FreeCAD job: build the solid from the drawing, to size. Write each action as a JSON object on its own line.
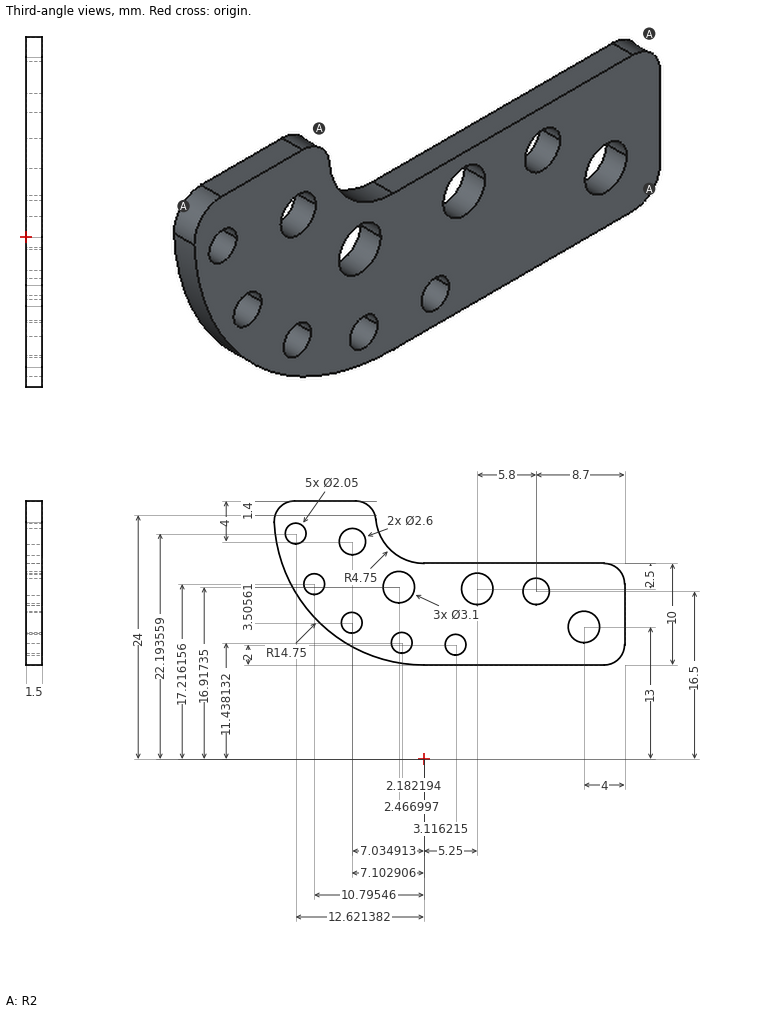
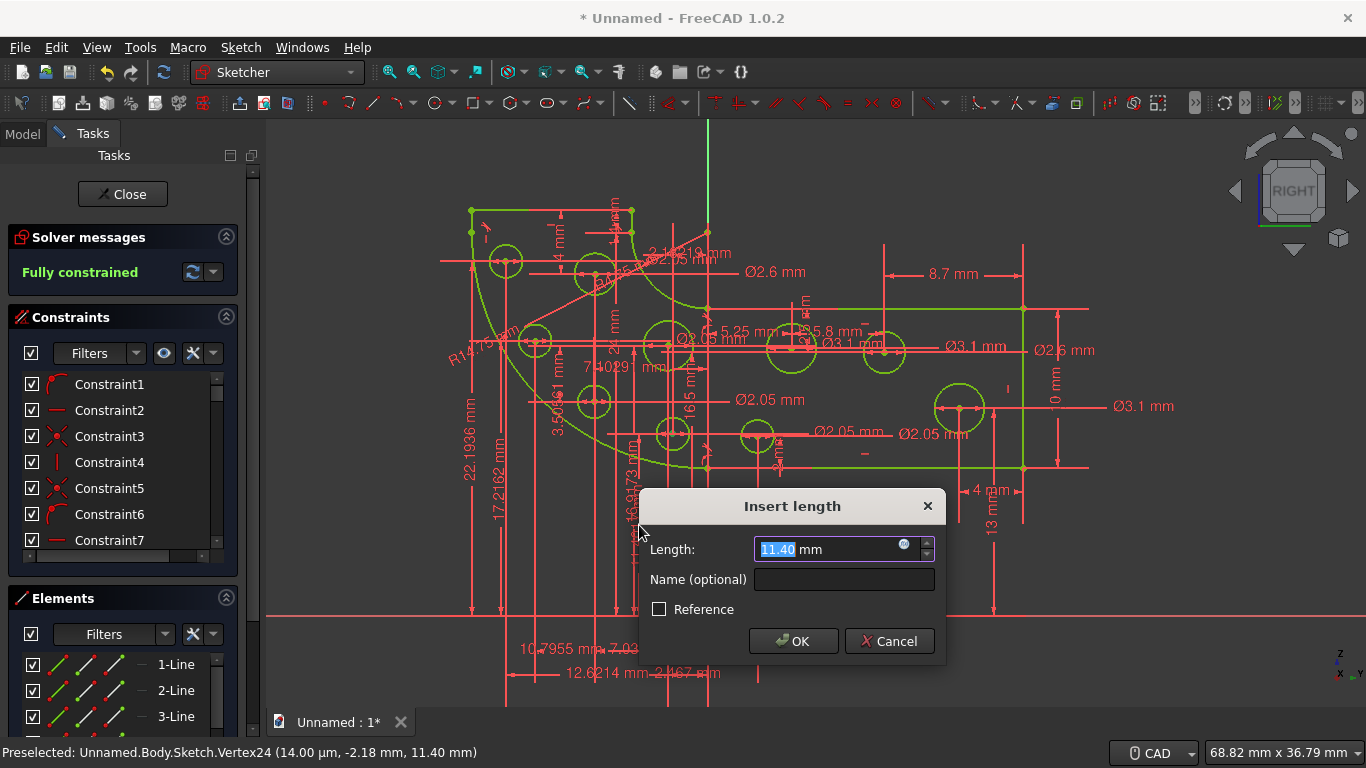
{"action": "type", "text": "11.438132"}
{"action": "key", "text": "Return"}
{"action": "key", "text": "Escape"}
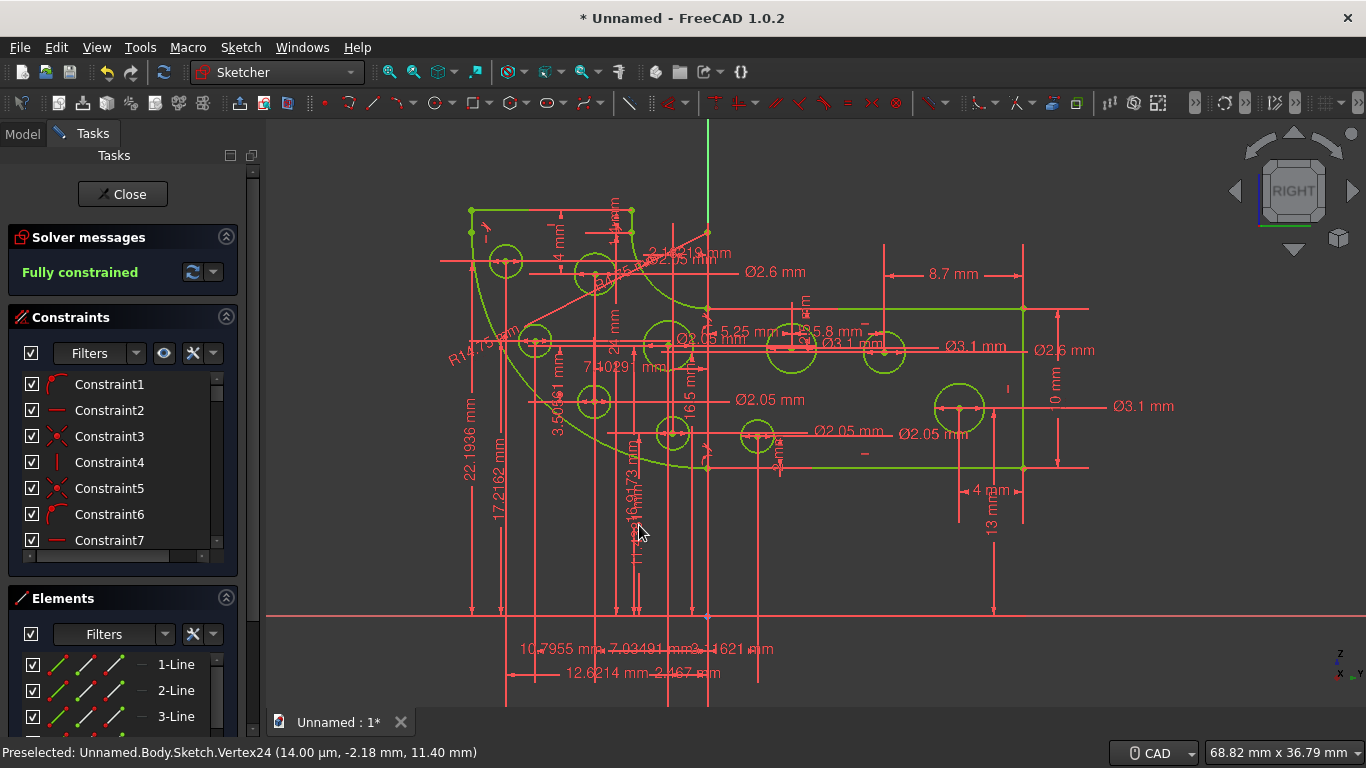
{"action": "left_click", "coordinate": [123, 194]}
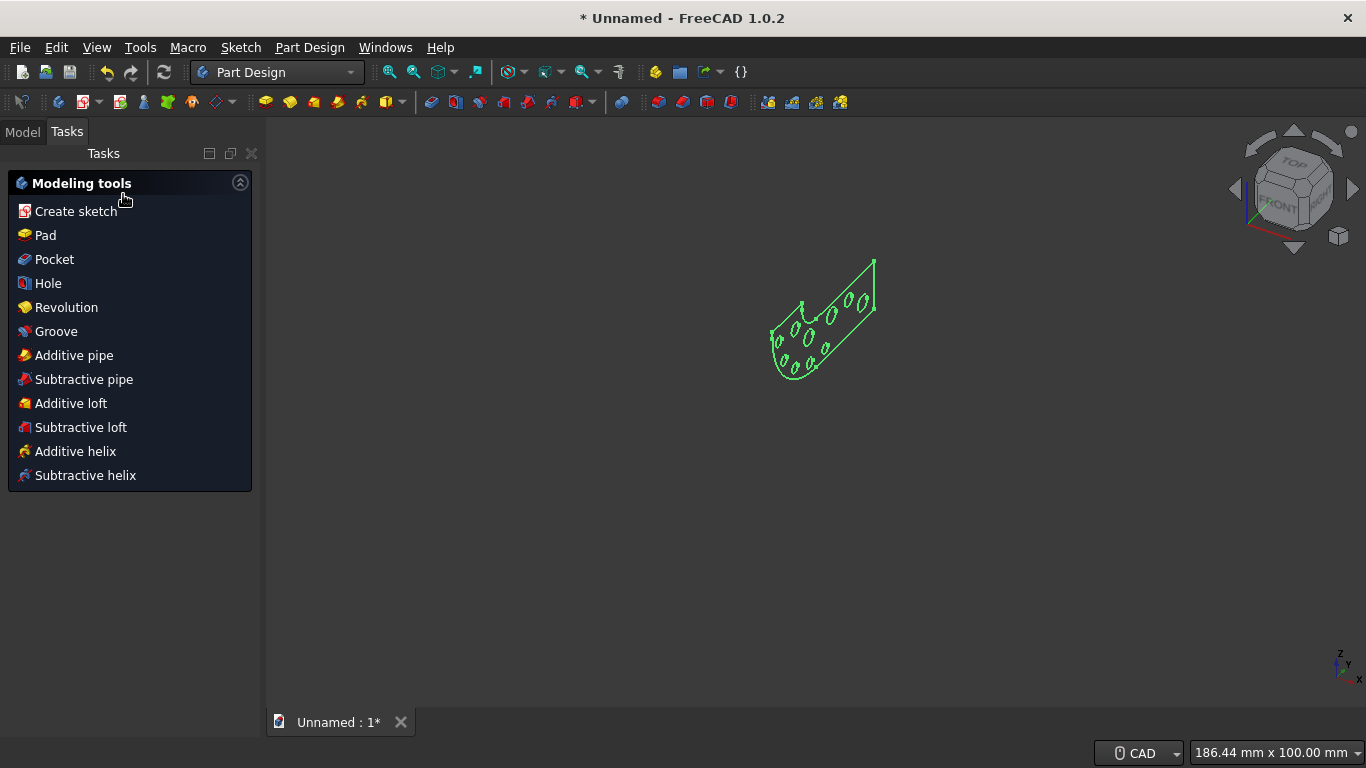
{"action": "left_click", "coordinate": [266, 102]}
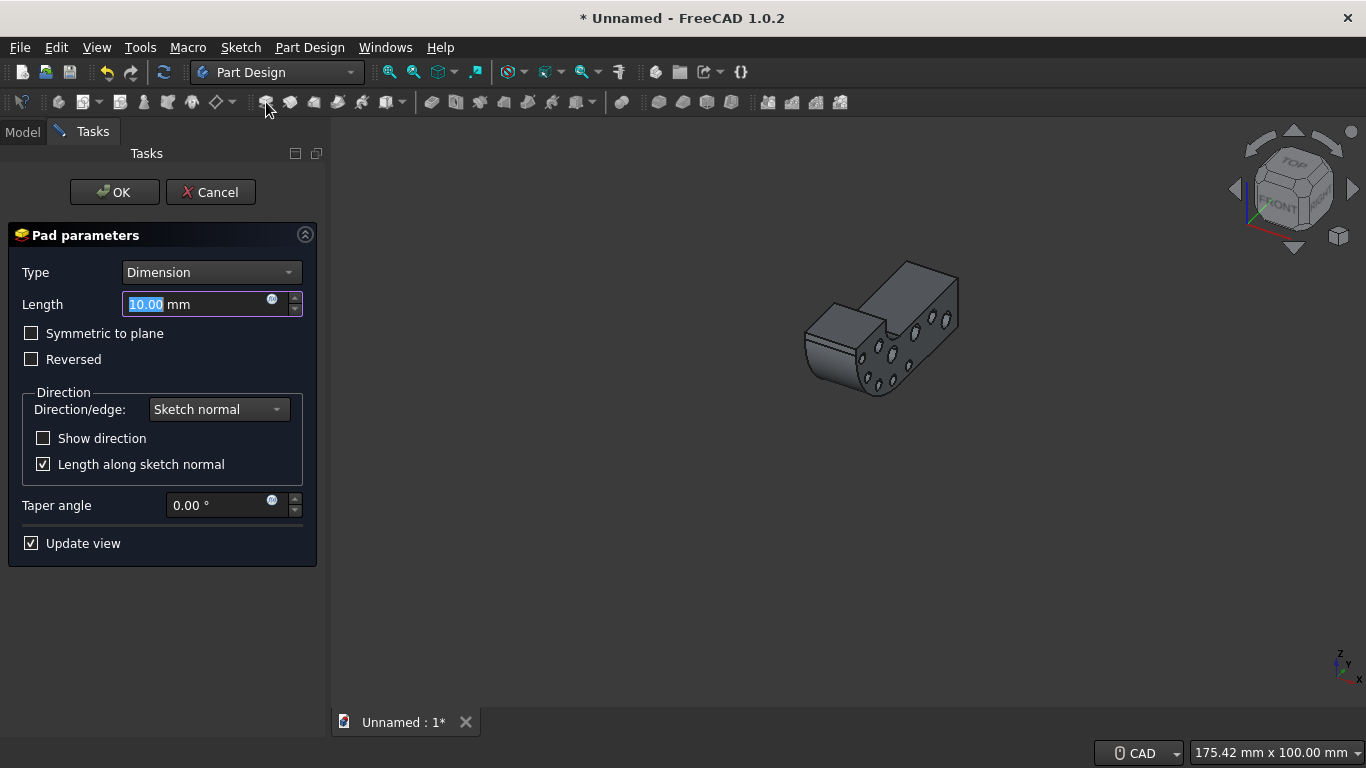
{"action": "type", "text": "1.5"}
{"action": "key", "text": "Tab"}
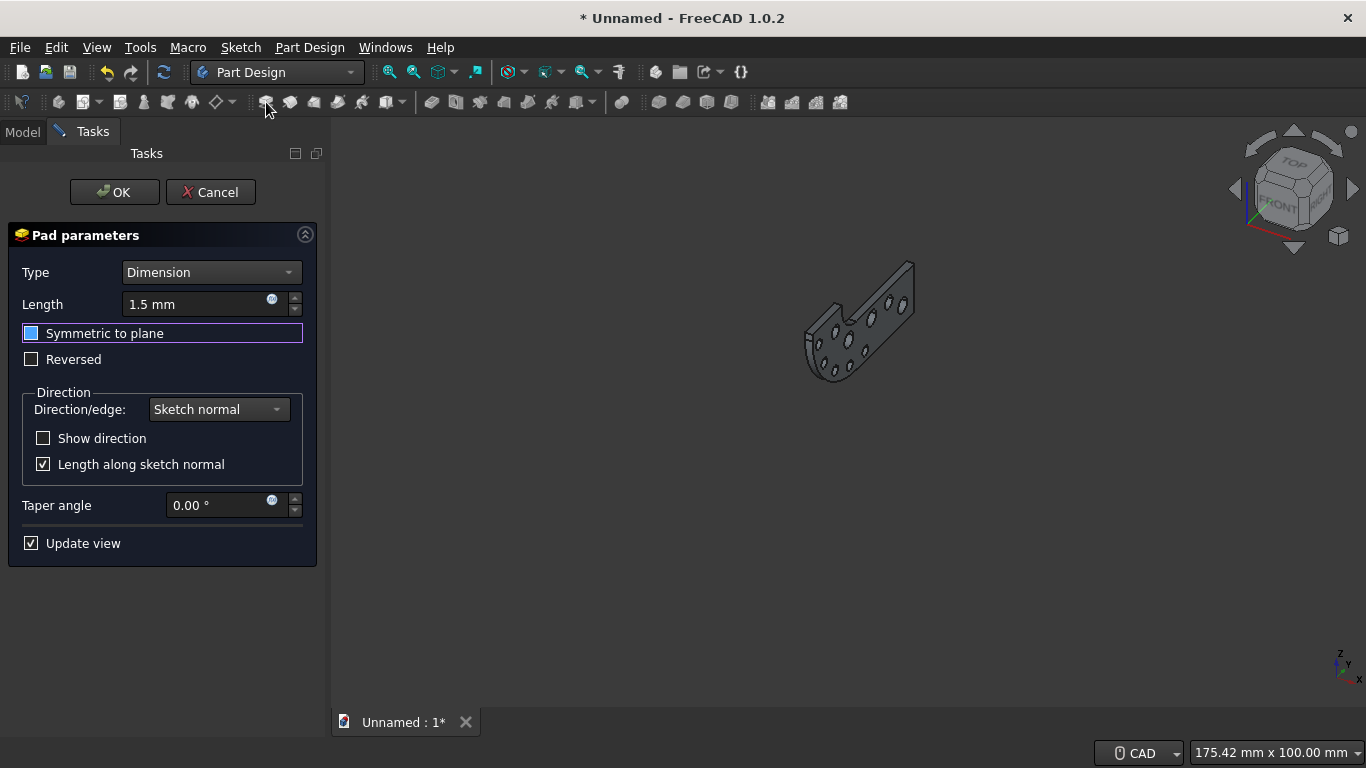
{"action": "left_click", "coordinate": [115, 192]}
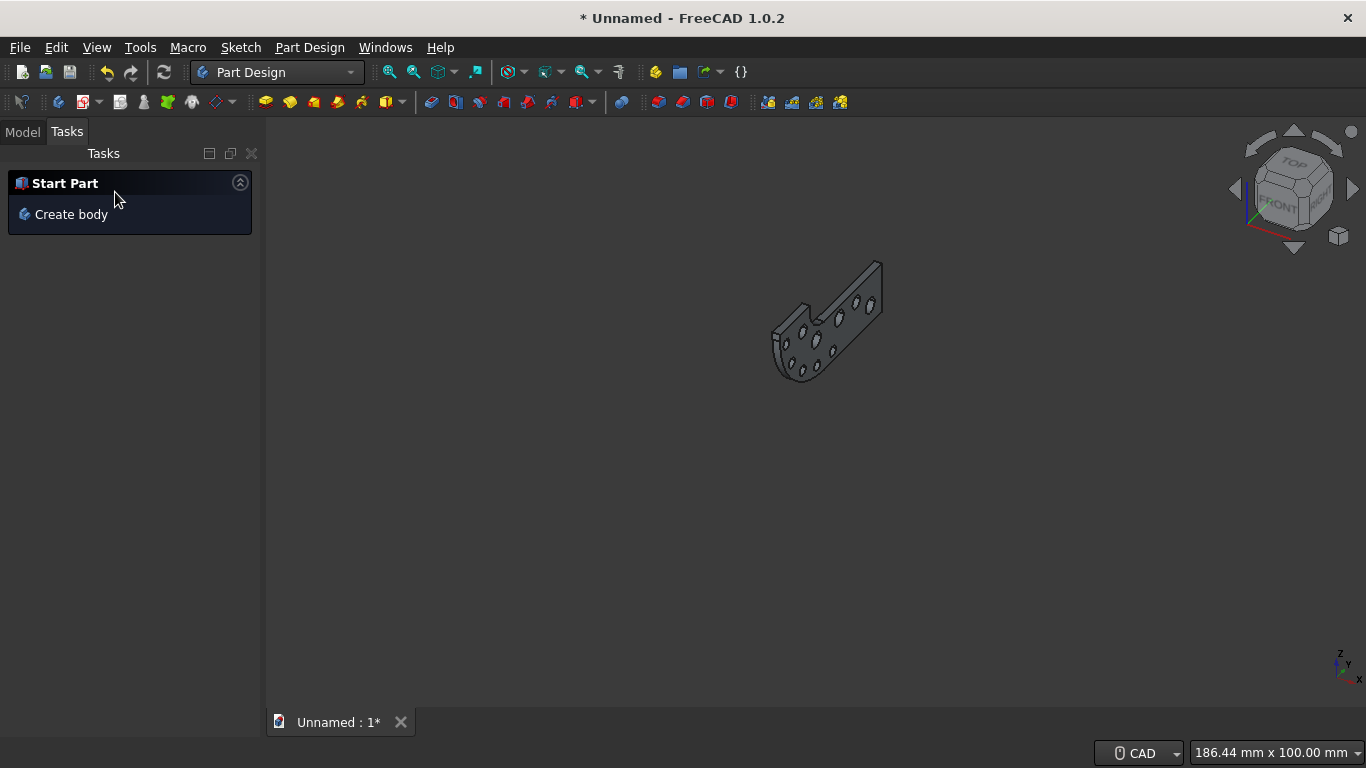
{"action": "key", "text": "v f"}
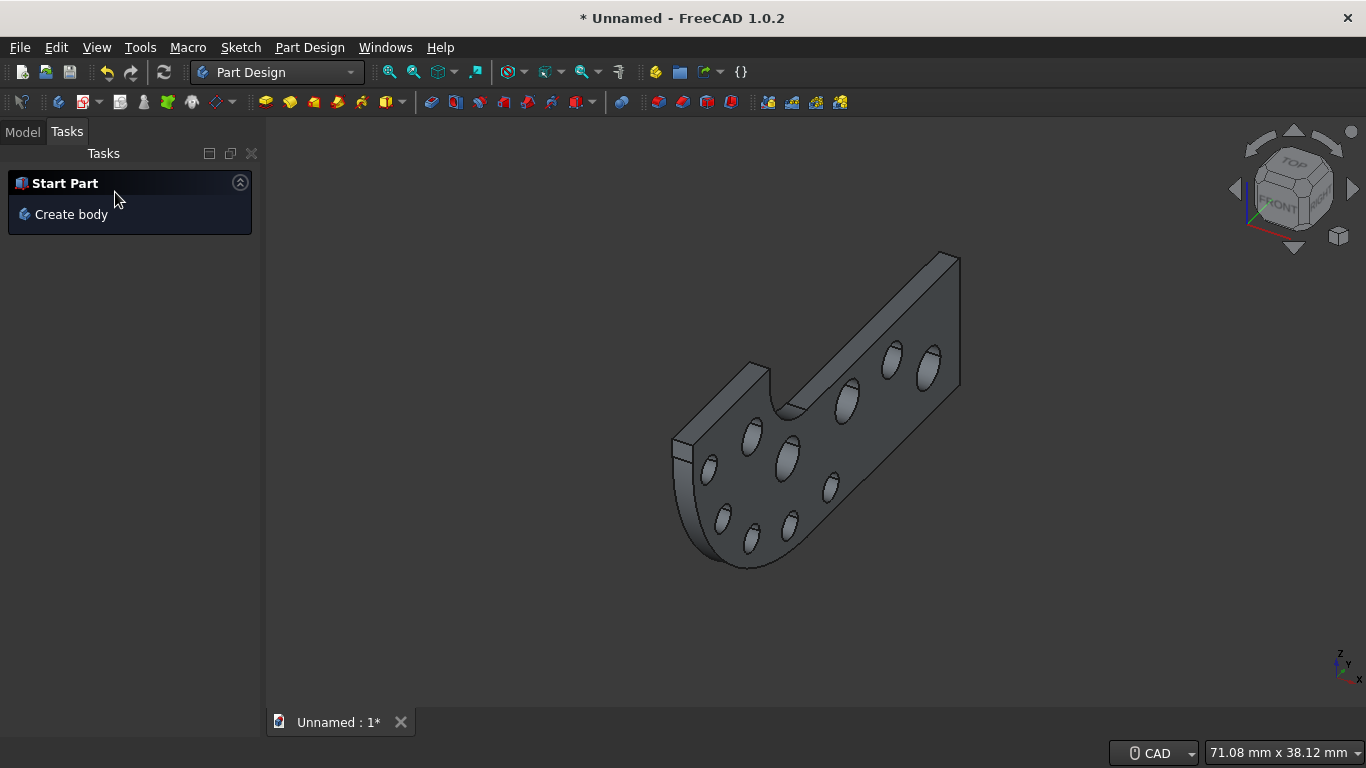
{"action": "left_click", "coordinate": [683, 441]}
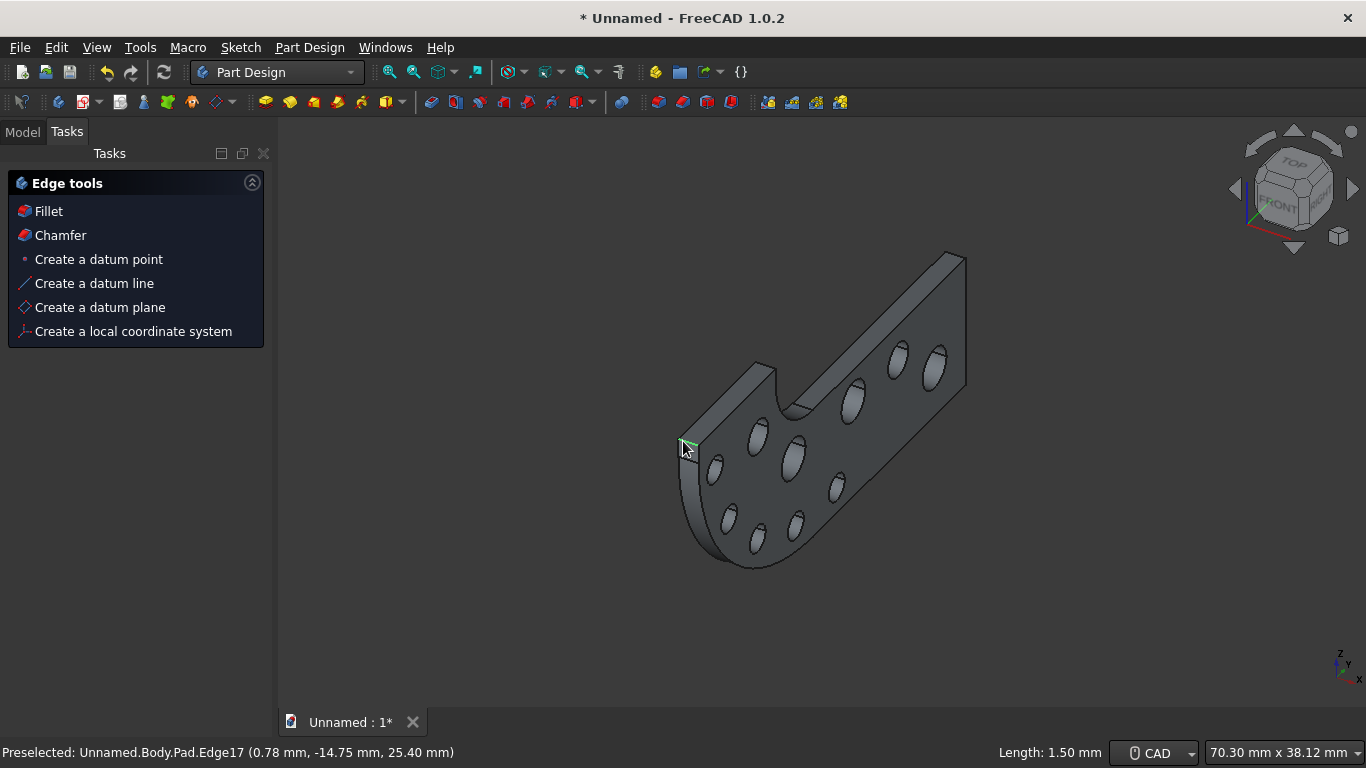
{"action": "key", "text": "0"}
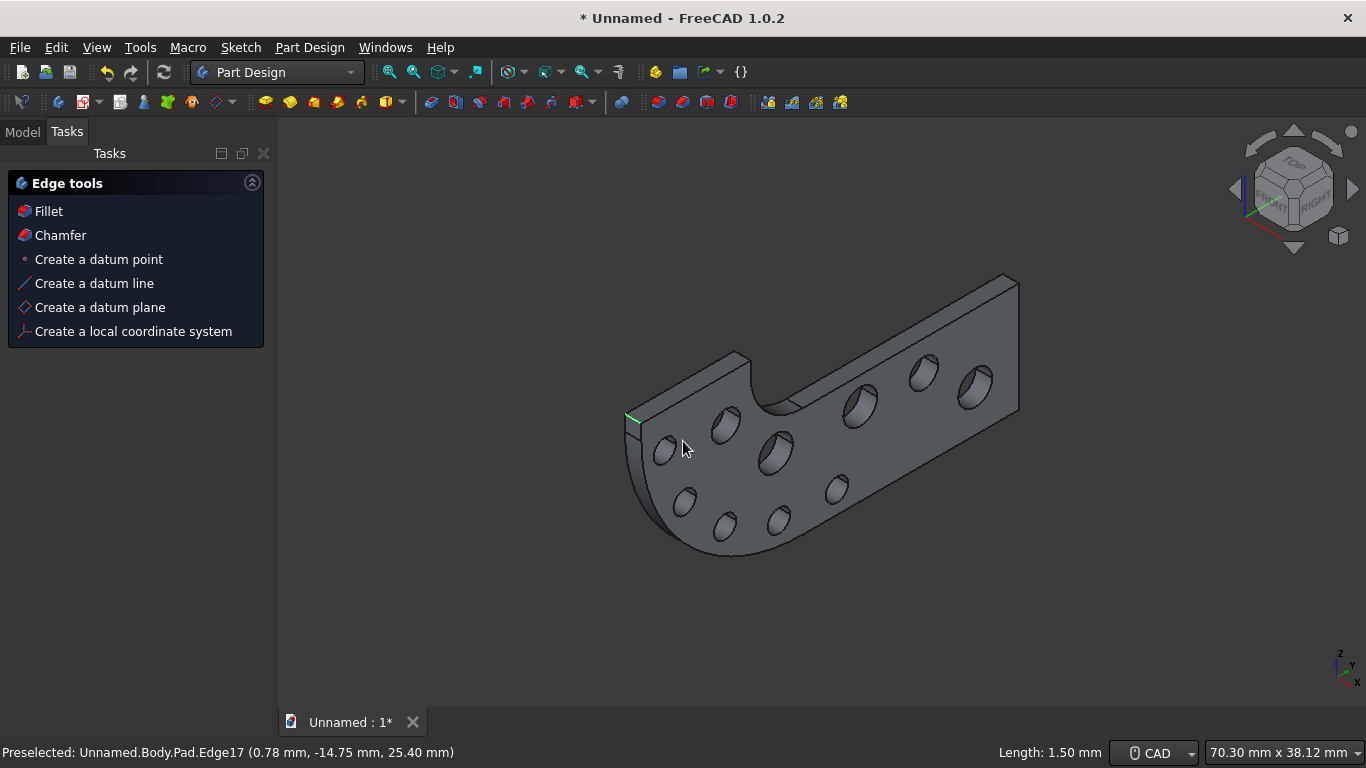
{"action": "key", "text": "2"}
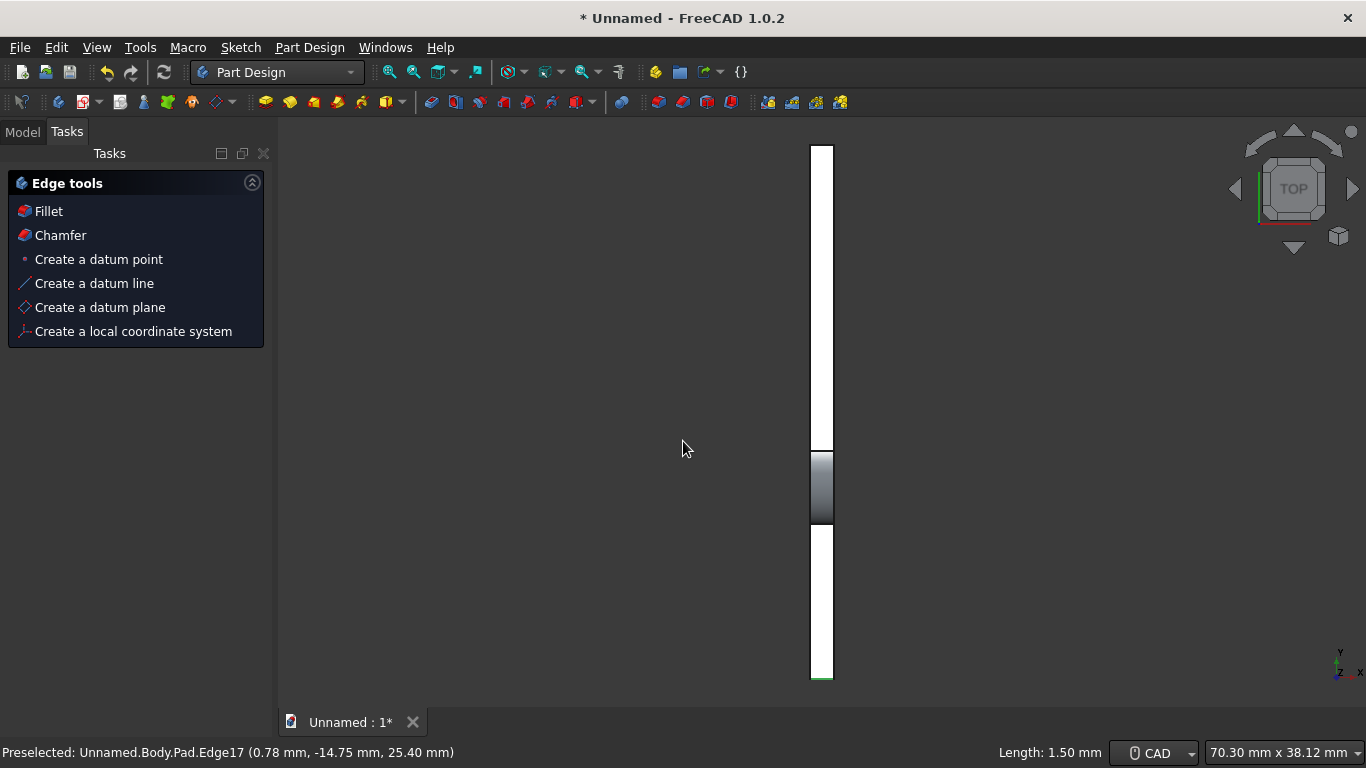
{"action": "left_click", "coordinate": [822, 523], "text": "ctrl"}